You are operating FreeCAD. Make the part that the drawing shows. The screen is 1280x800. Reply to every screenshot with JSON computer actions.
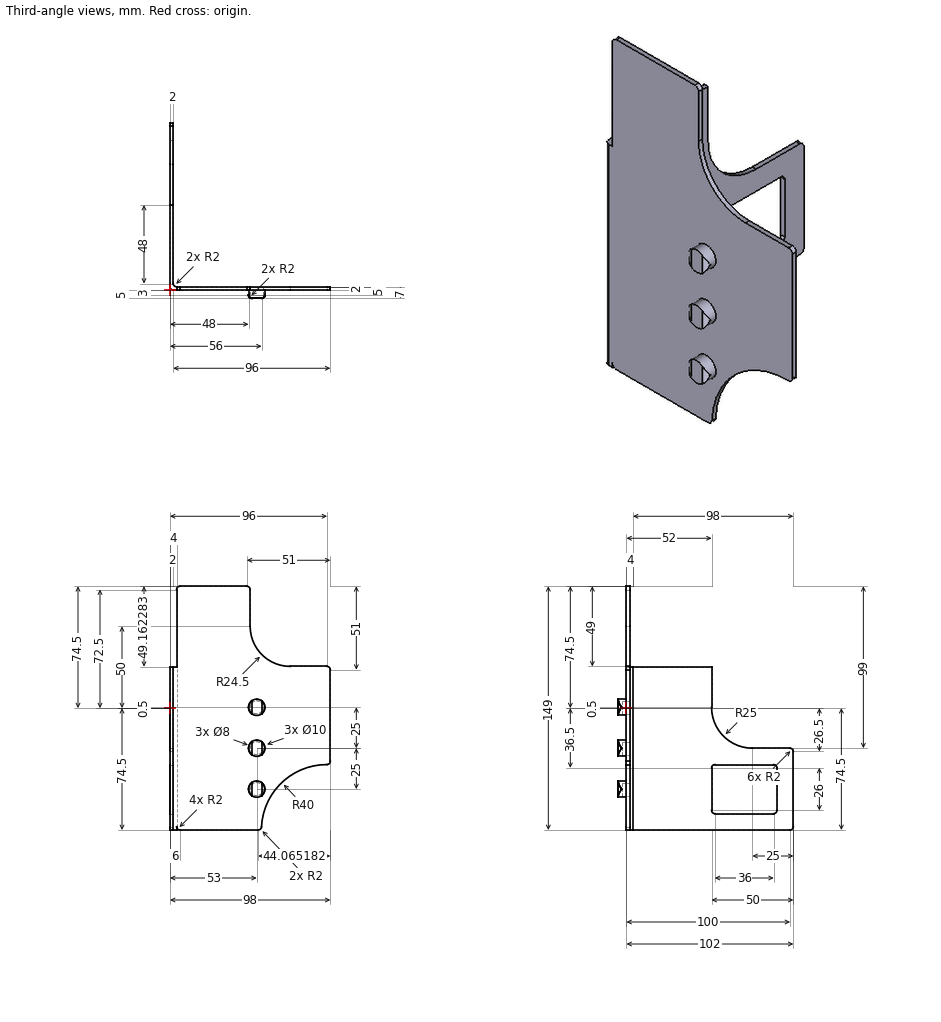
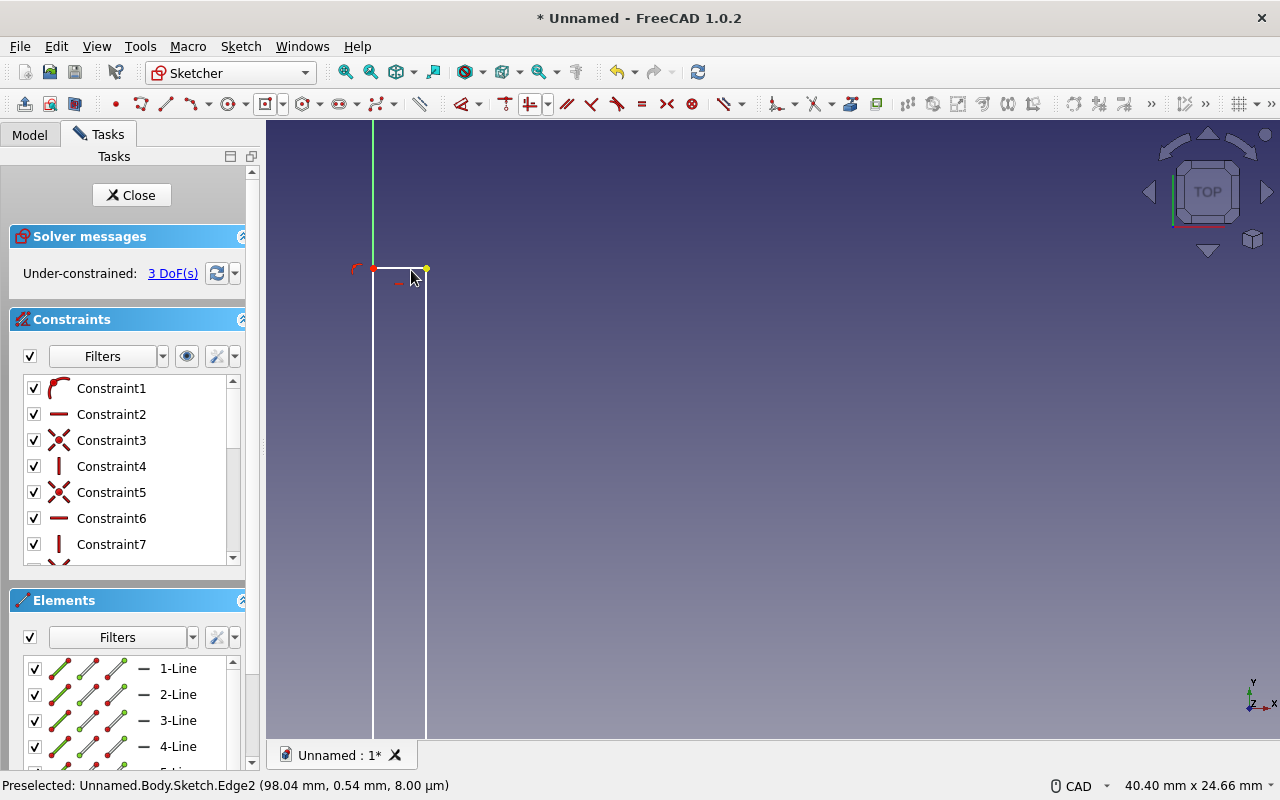
{"action": "left_click", "coordinate": [410, 268]}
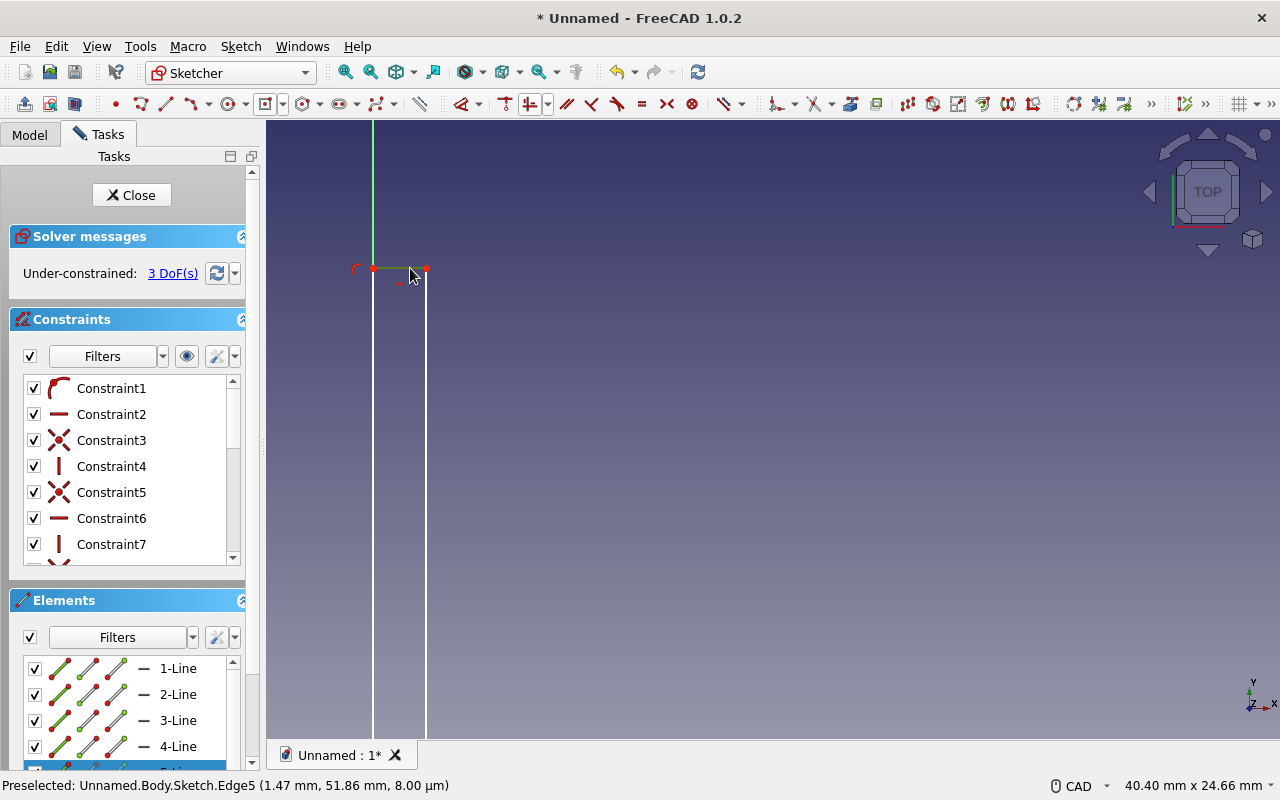
{"action": "key", "text": "l"}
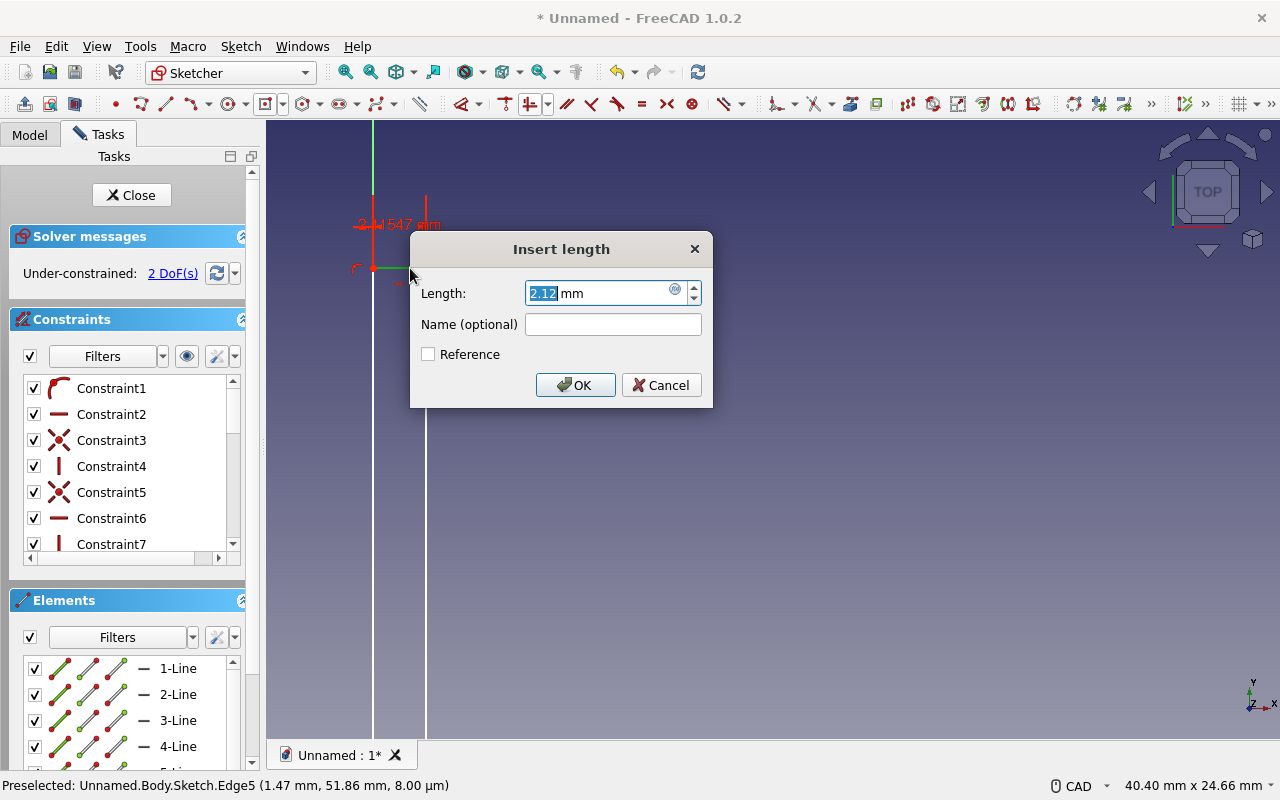
{"action": "type", "text": "2"}
{"action": "key", "text": "Return"}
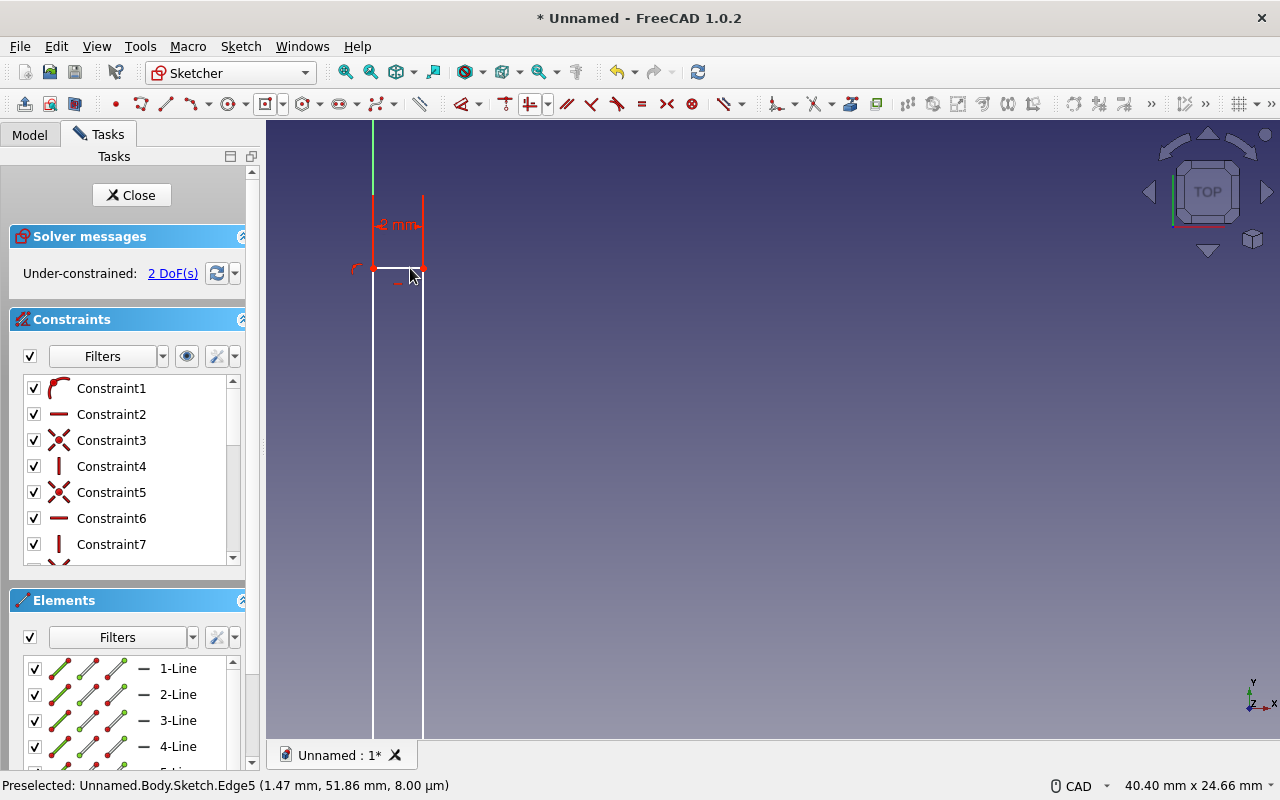
{"action": "scroll", "coordinate": [410, 270], "scroll_direction": "down", "scroll_amount": 7}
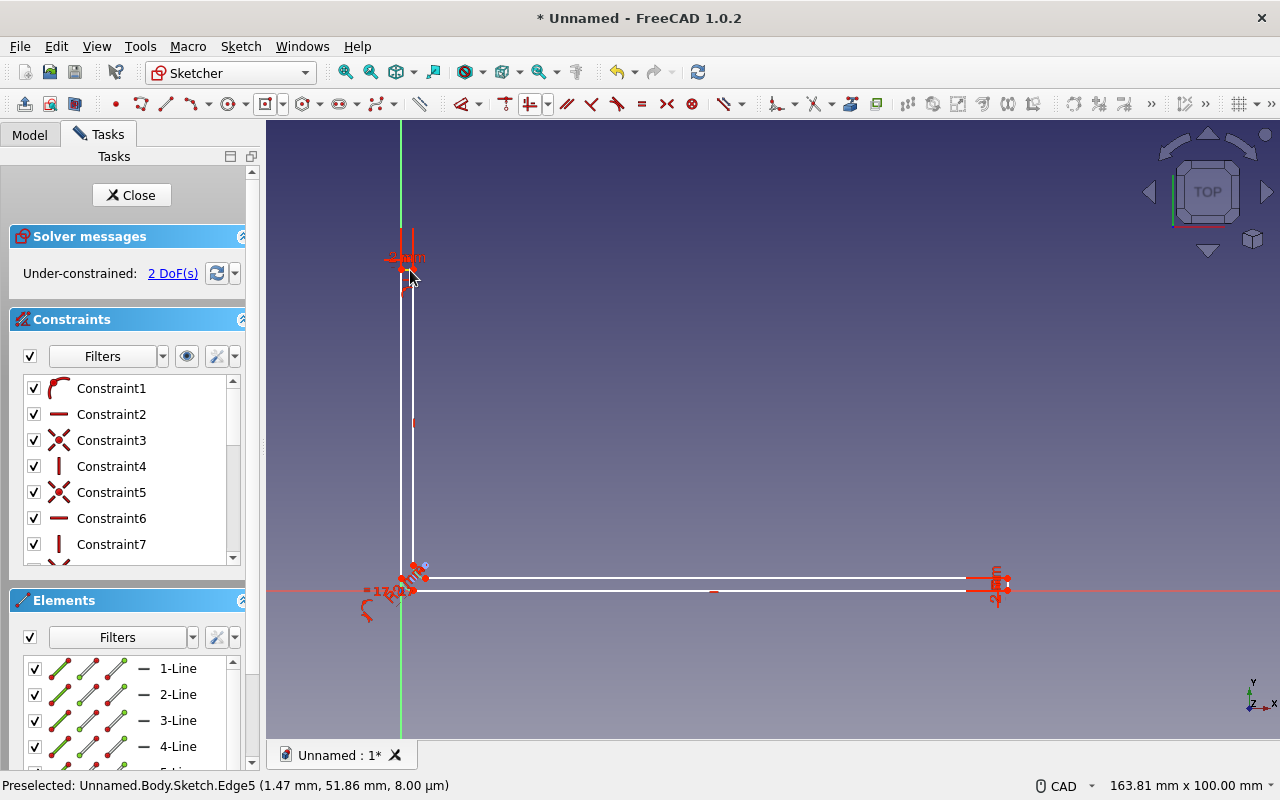
{"action": "left_click", "coordinate": [592, 591]}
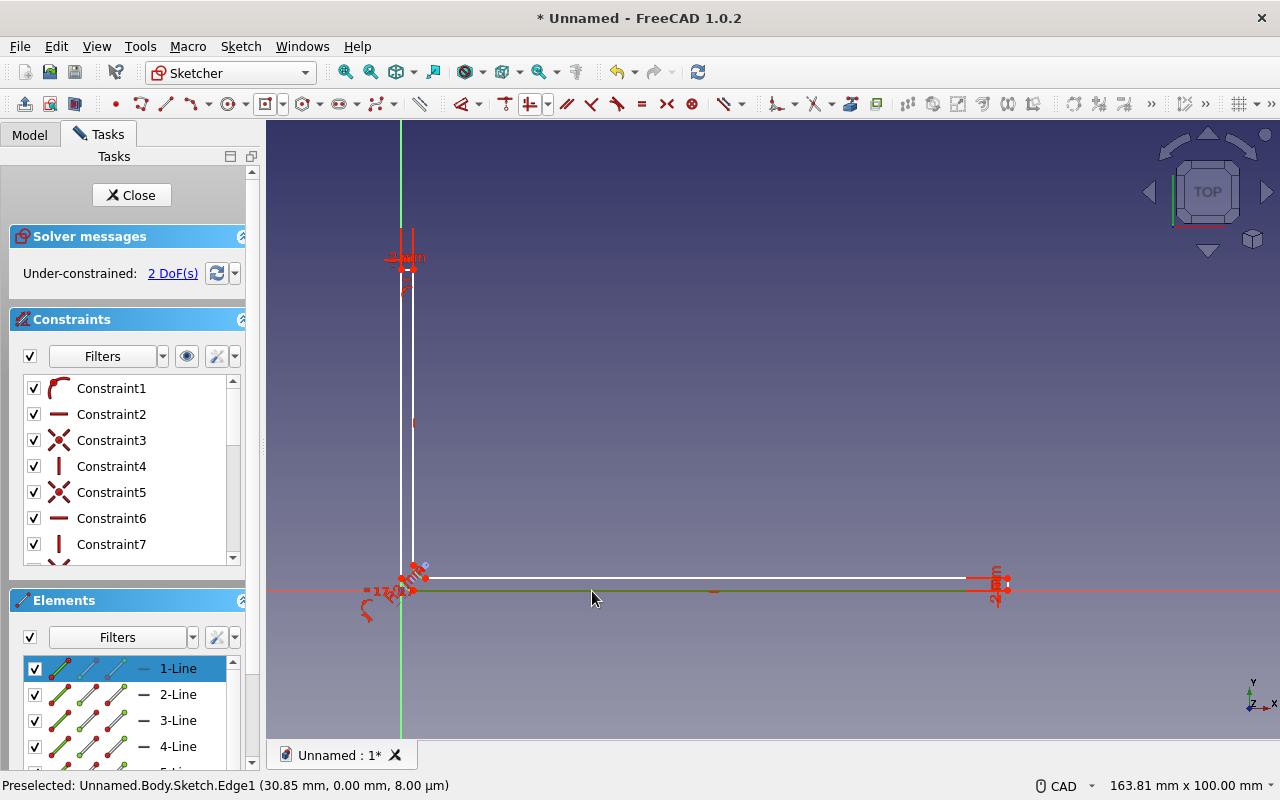
{"action": "key", "text": "l"}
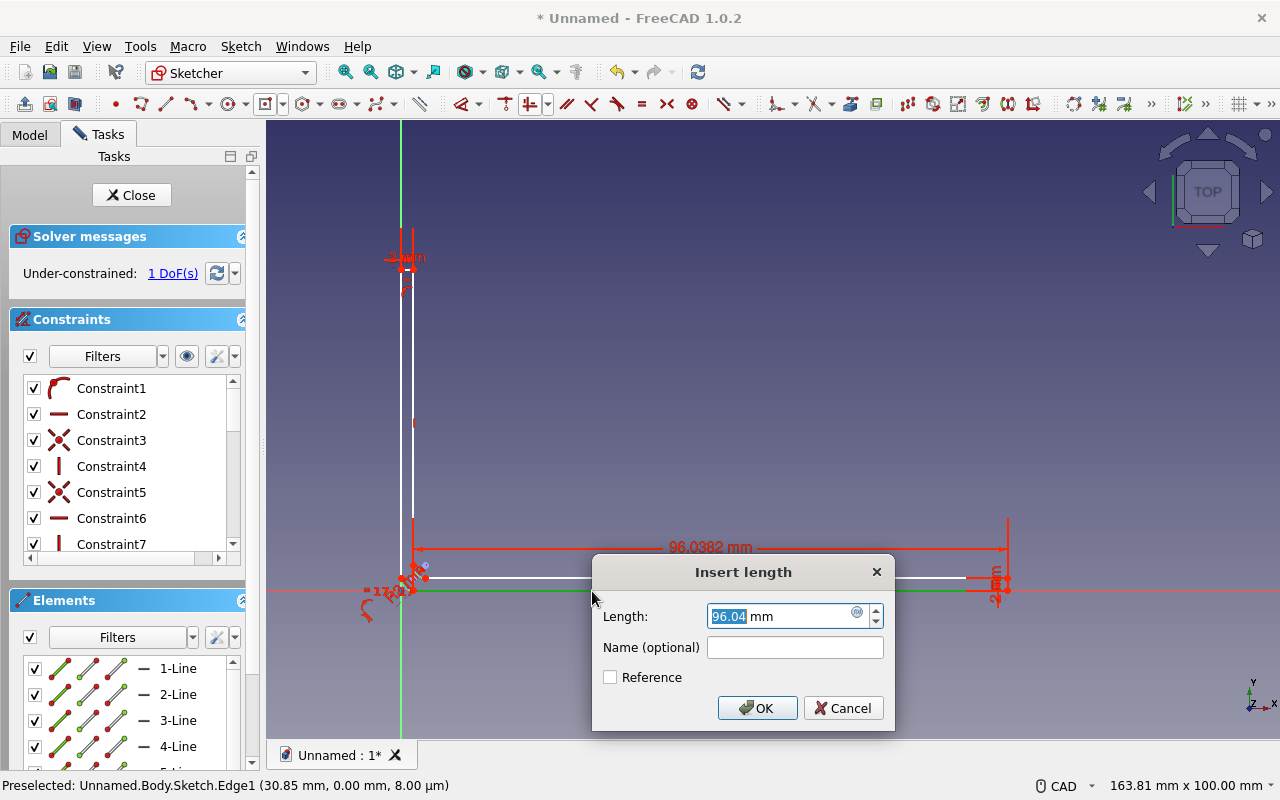
{"action": "type", "text": "96"}
{"action": "key", "text": "Return"}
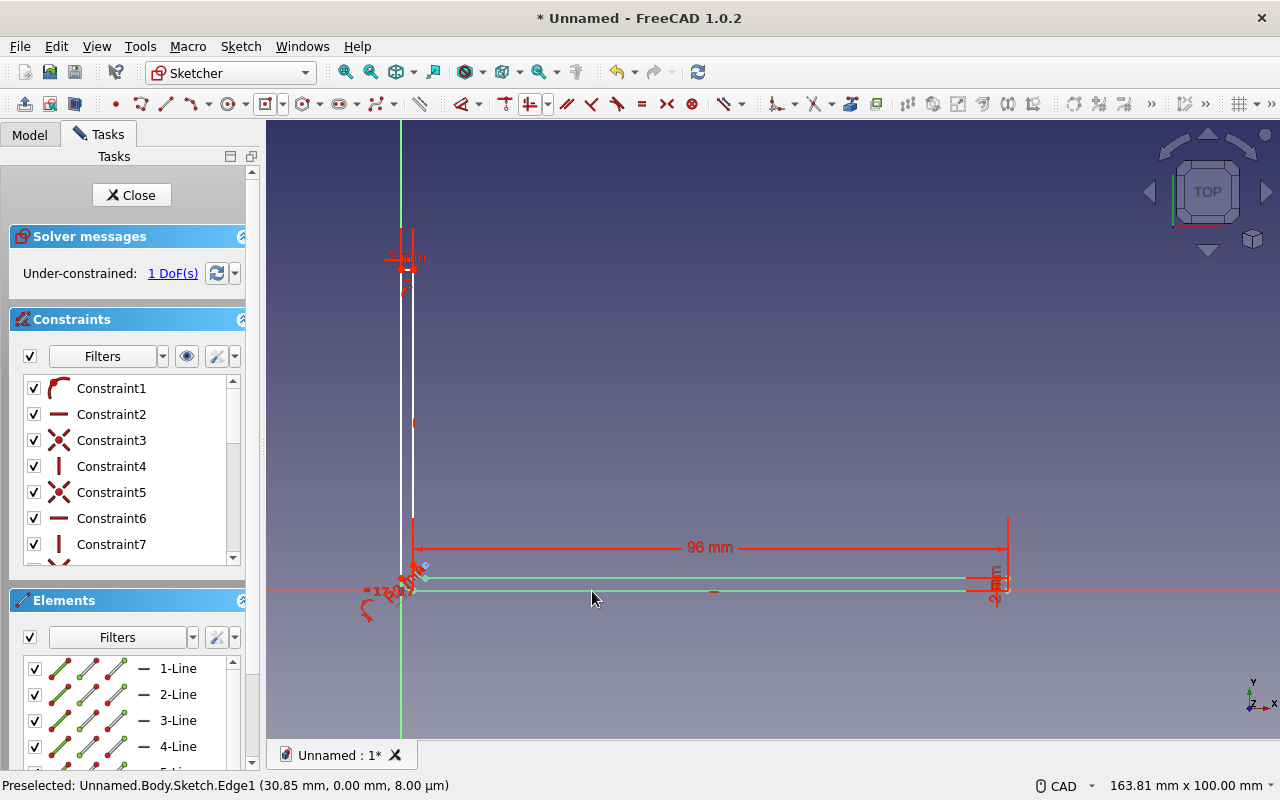
{"action": "left_click", "coordinate": [413, 477]}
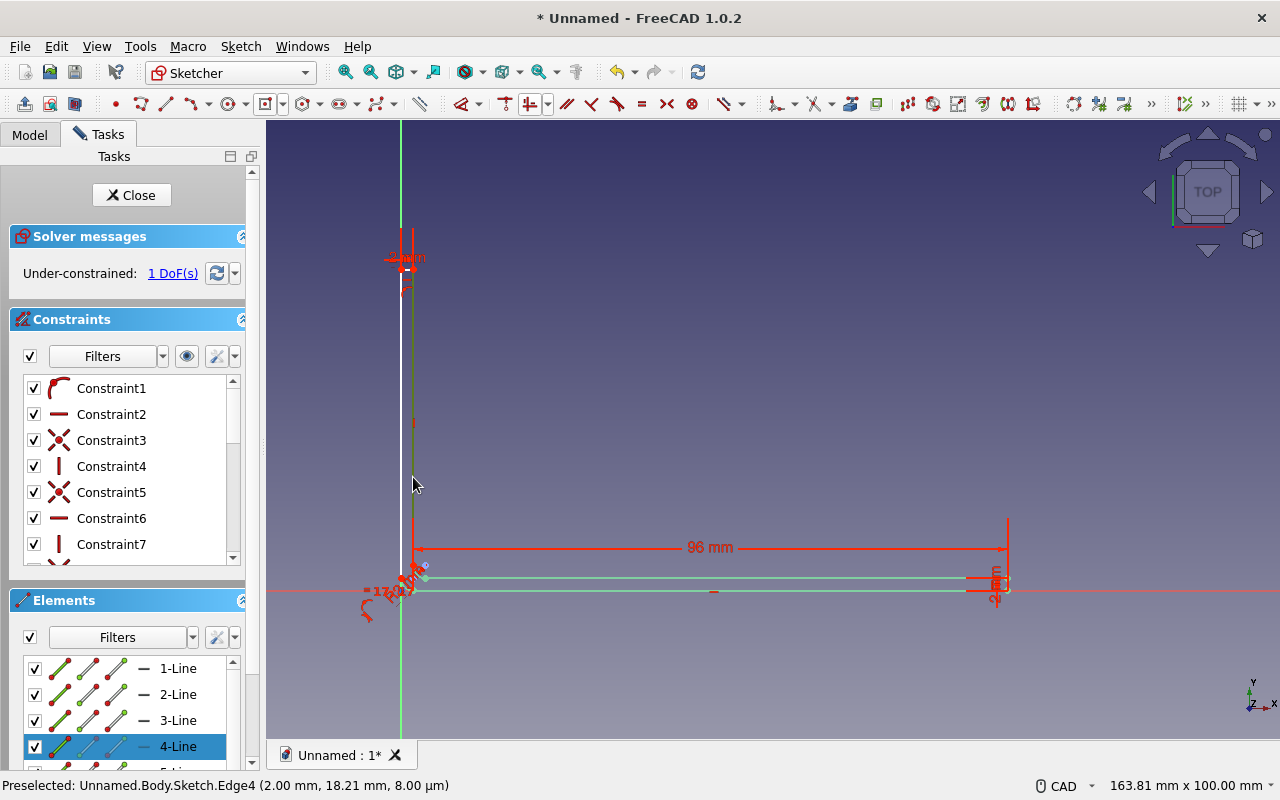
{"action": "key", "text": "i"}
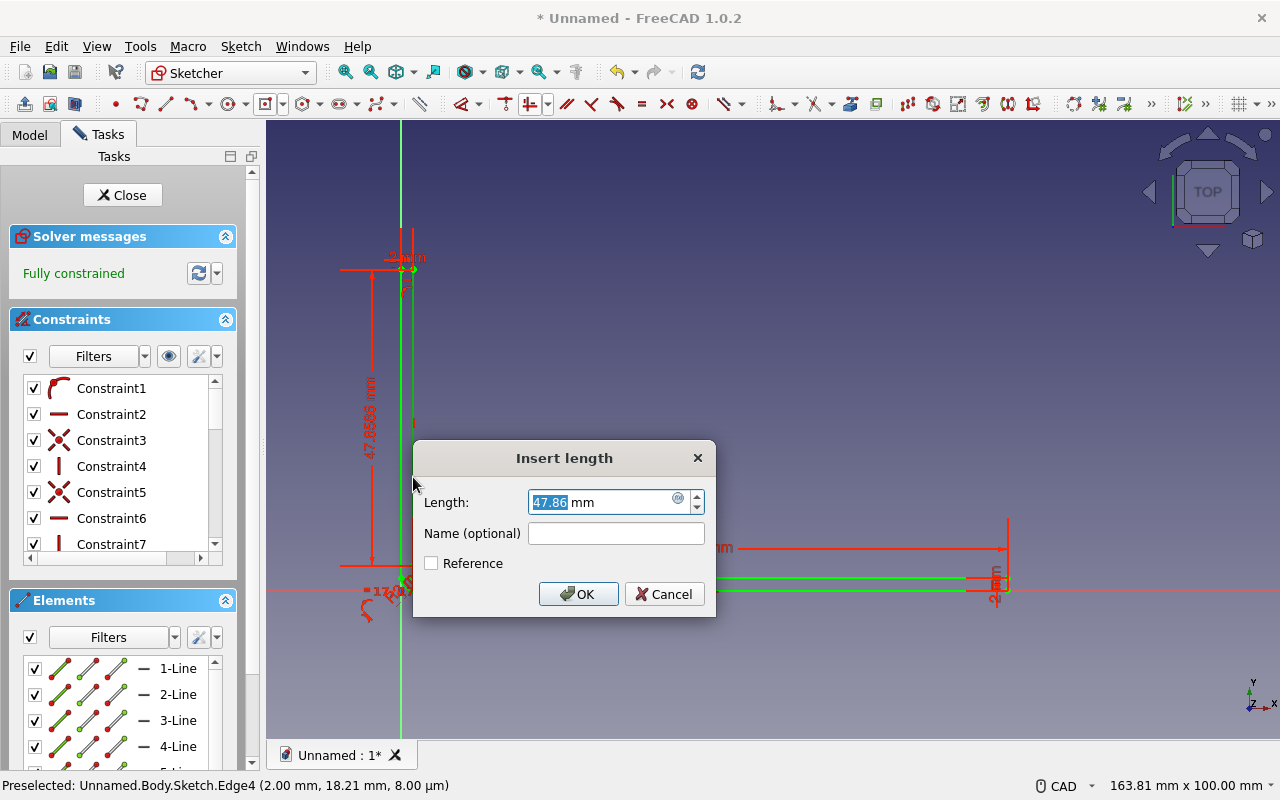
{"action": "type", "text": "48"}
{"action": "key", "text": "Return"}